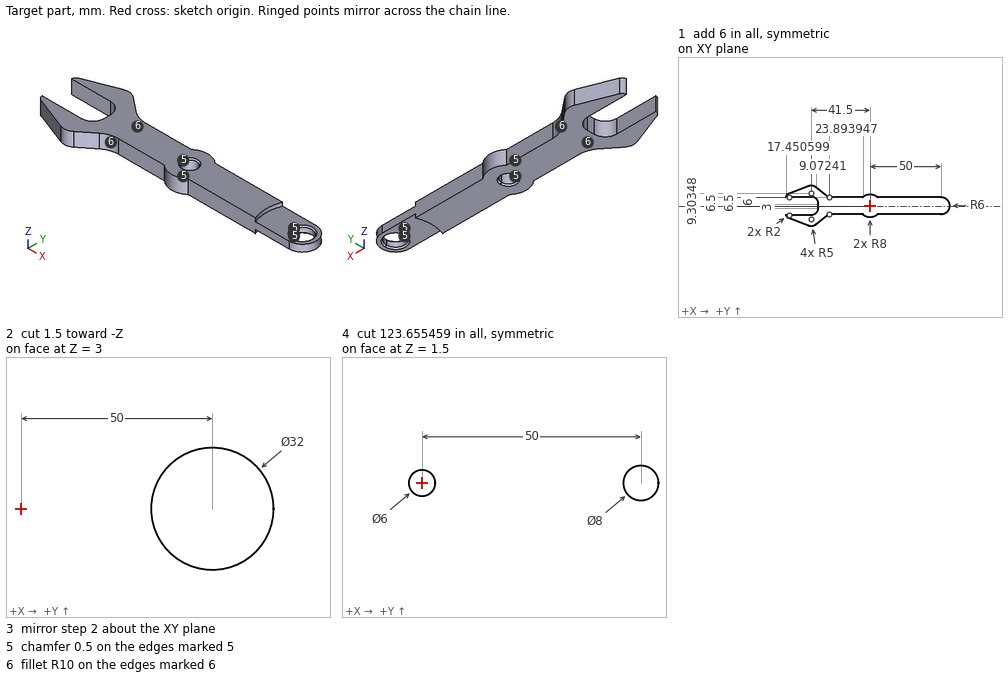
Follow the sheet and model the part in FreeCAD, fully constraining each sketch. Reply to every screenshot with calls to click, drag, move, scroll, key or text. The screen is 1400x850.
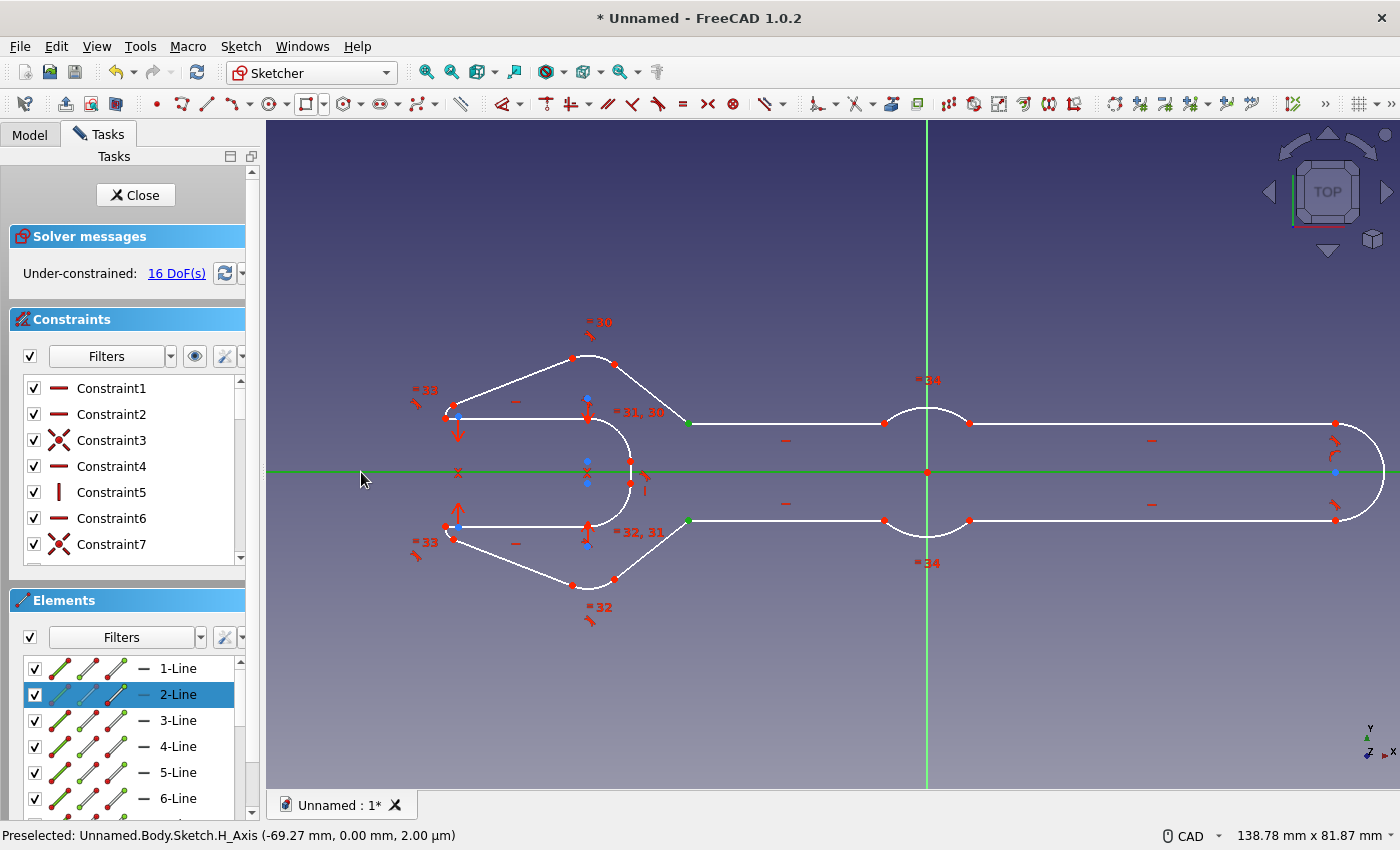
click(708, 104)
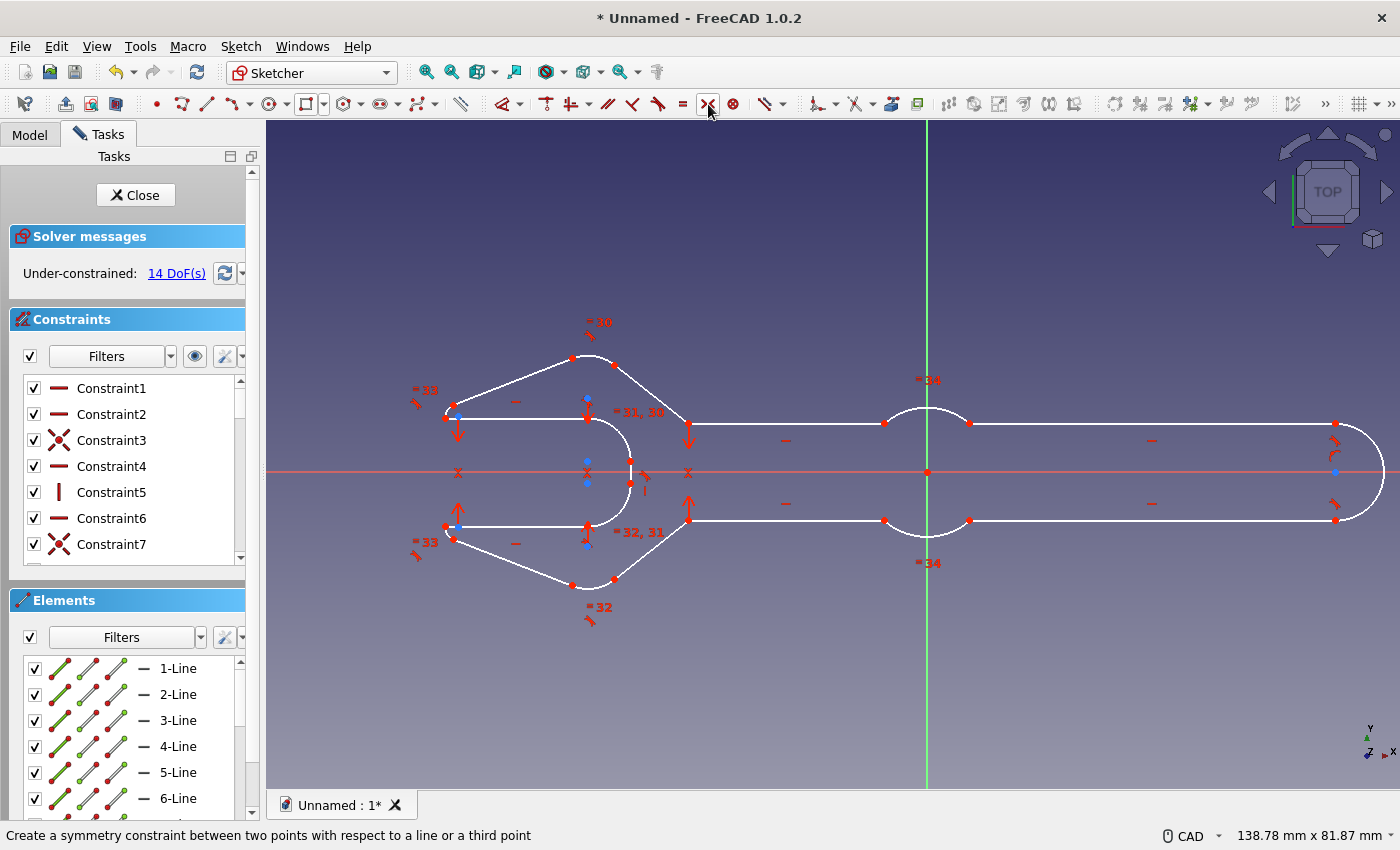
click(502, 104)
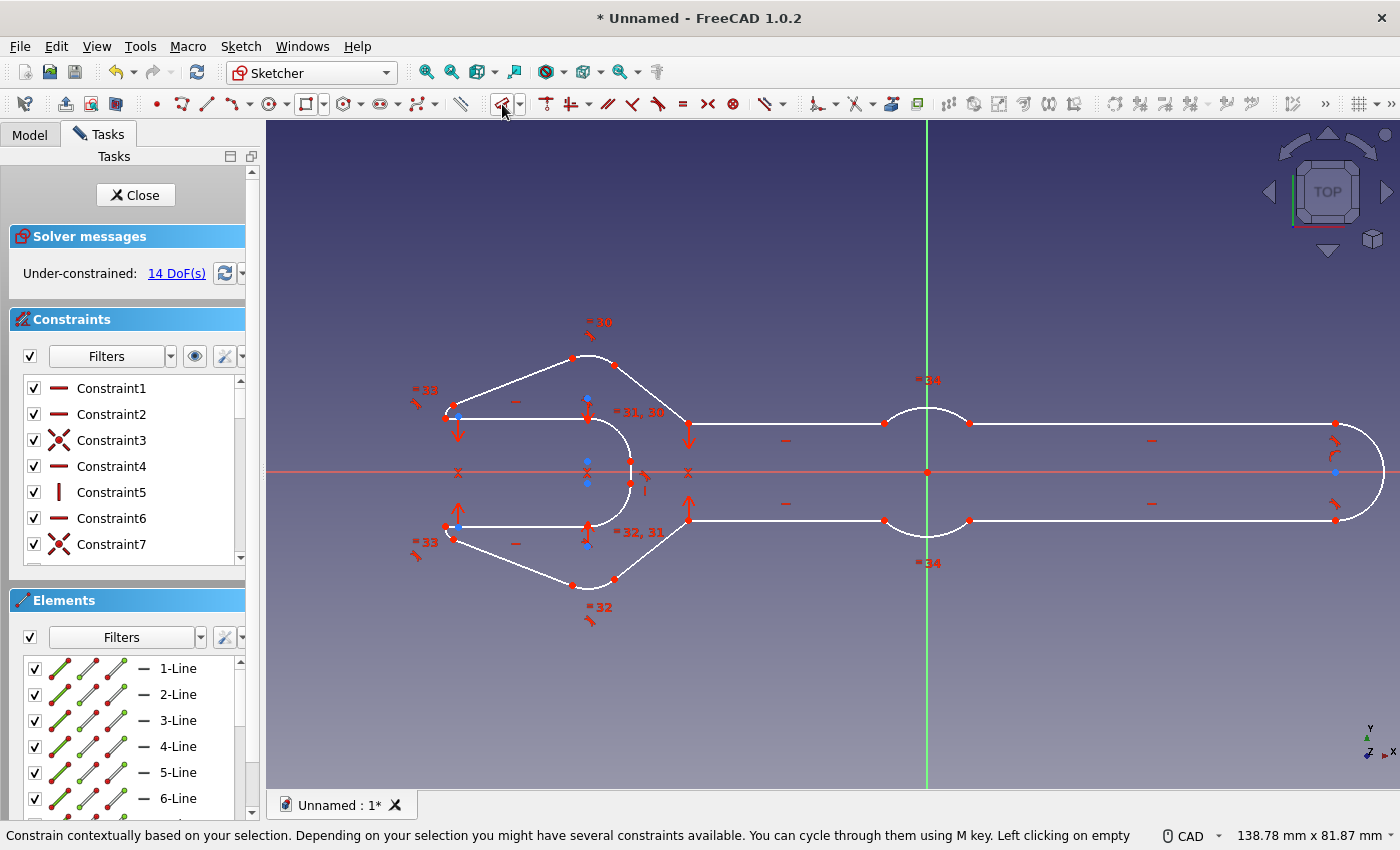
click(945, 410)
click(954, 379)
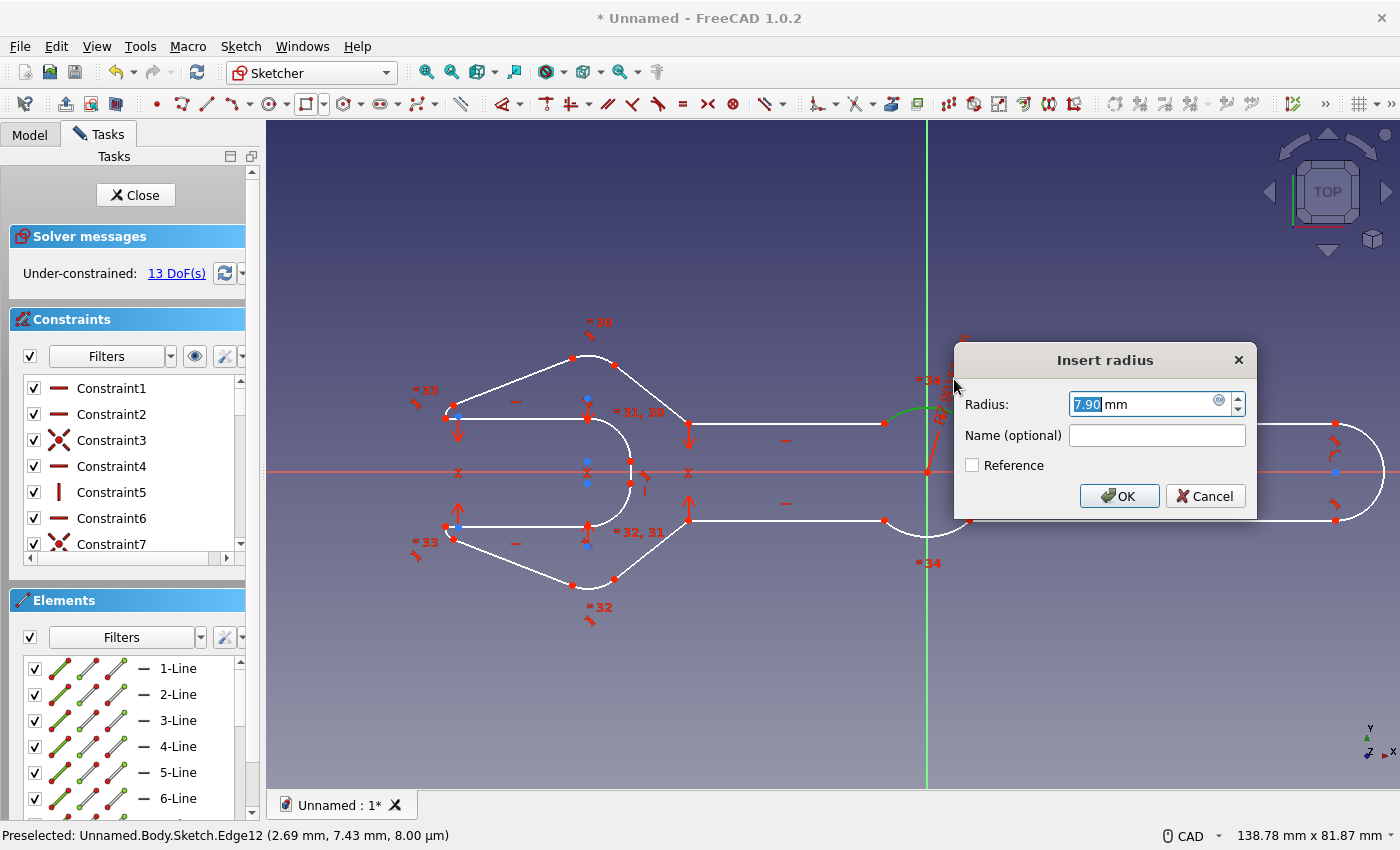
text(8)
key(Return)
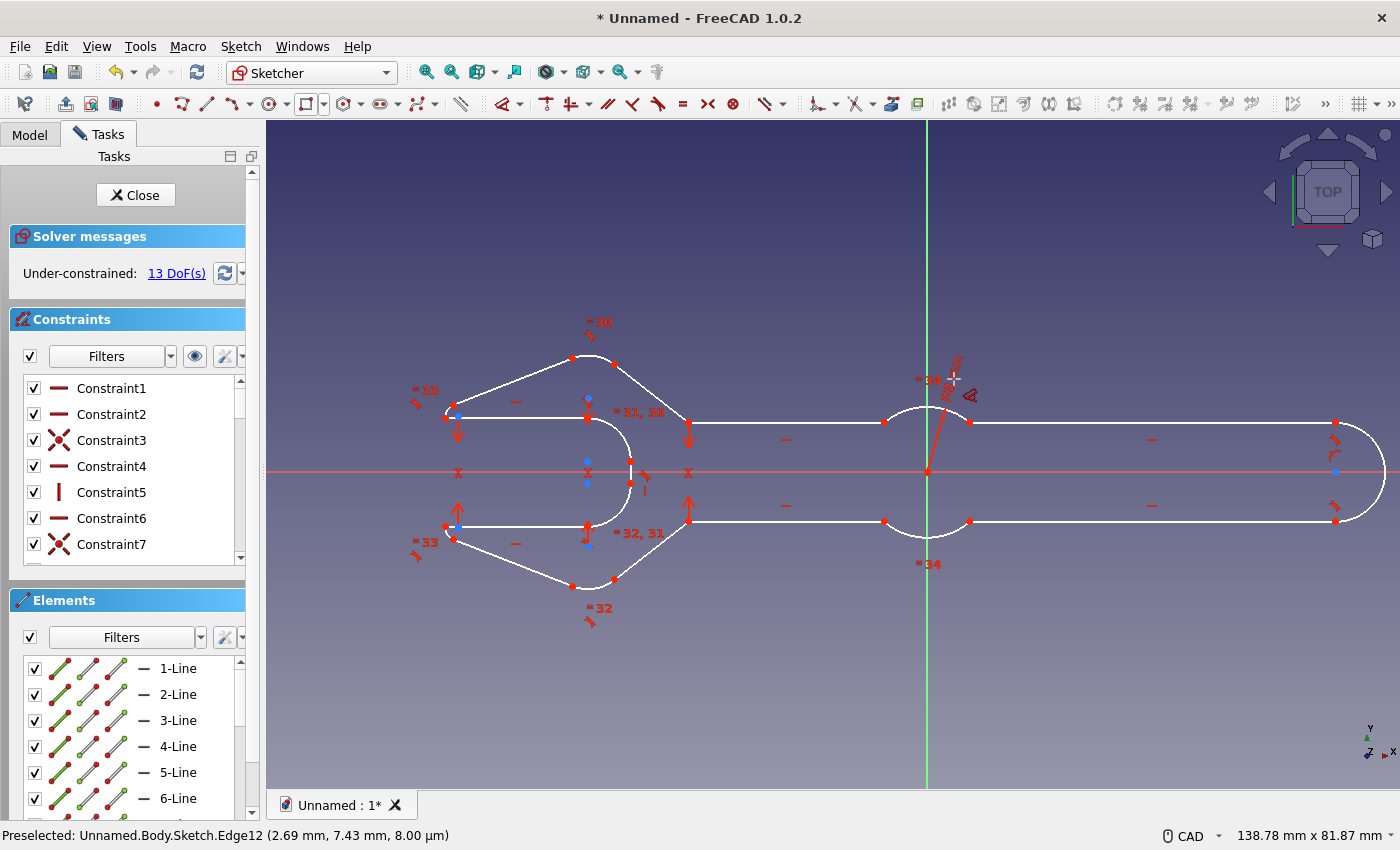
click(603, 358)
click(614, 328)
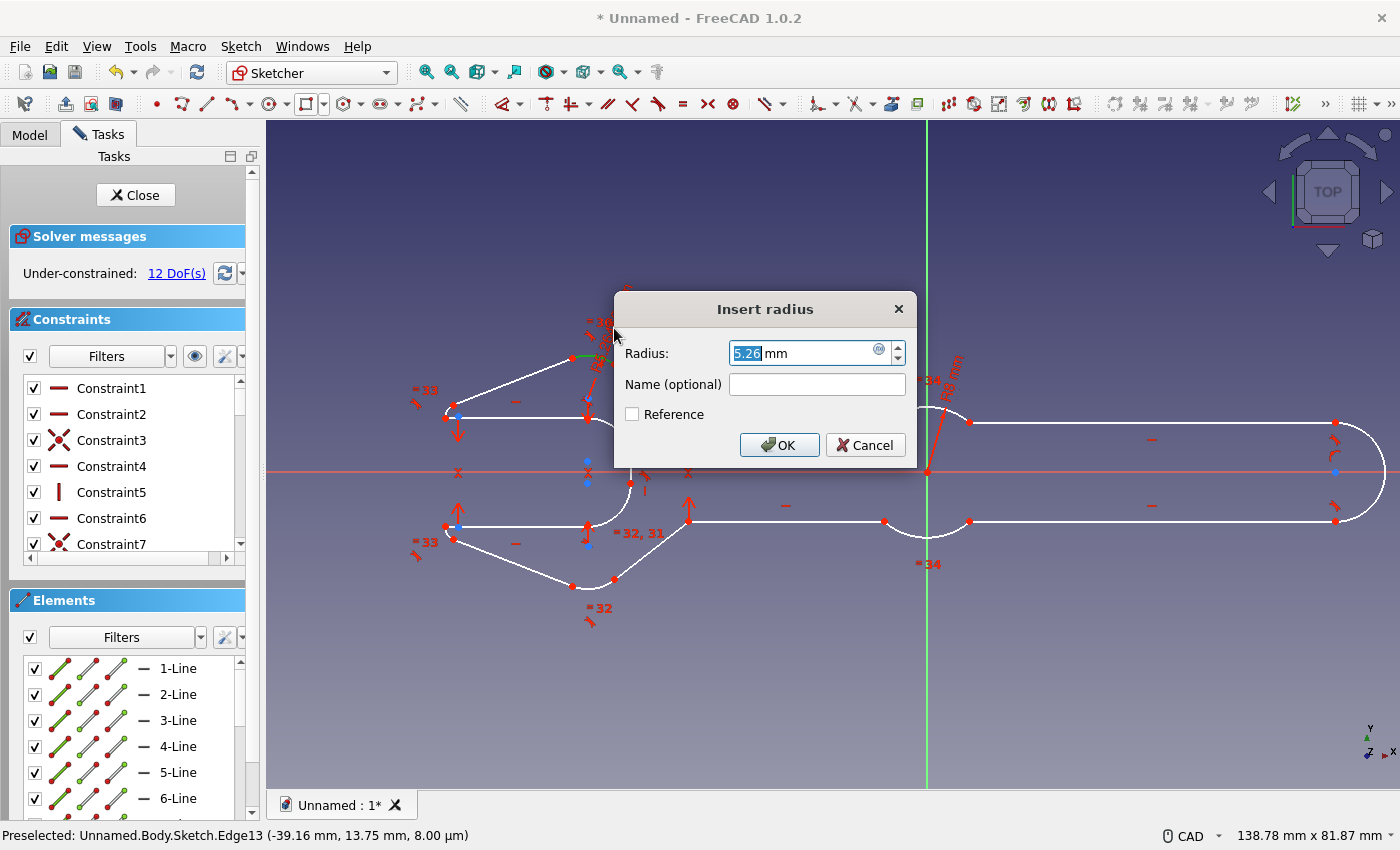
text(5)
key(Return)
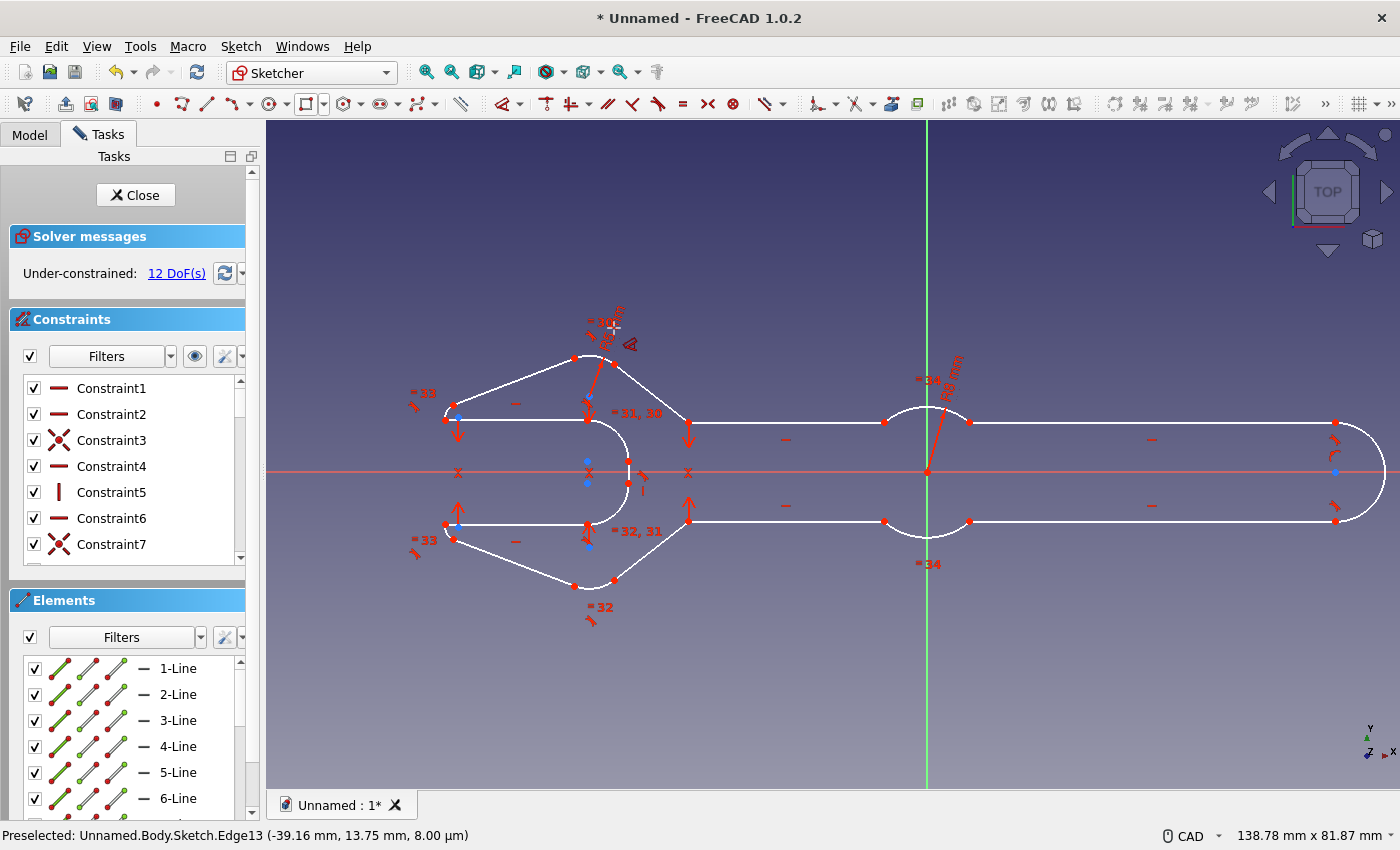
scroll(447, 411, up, 5)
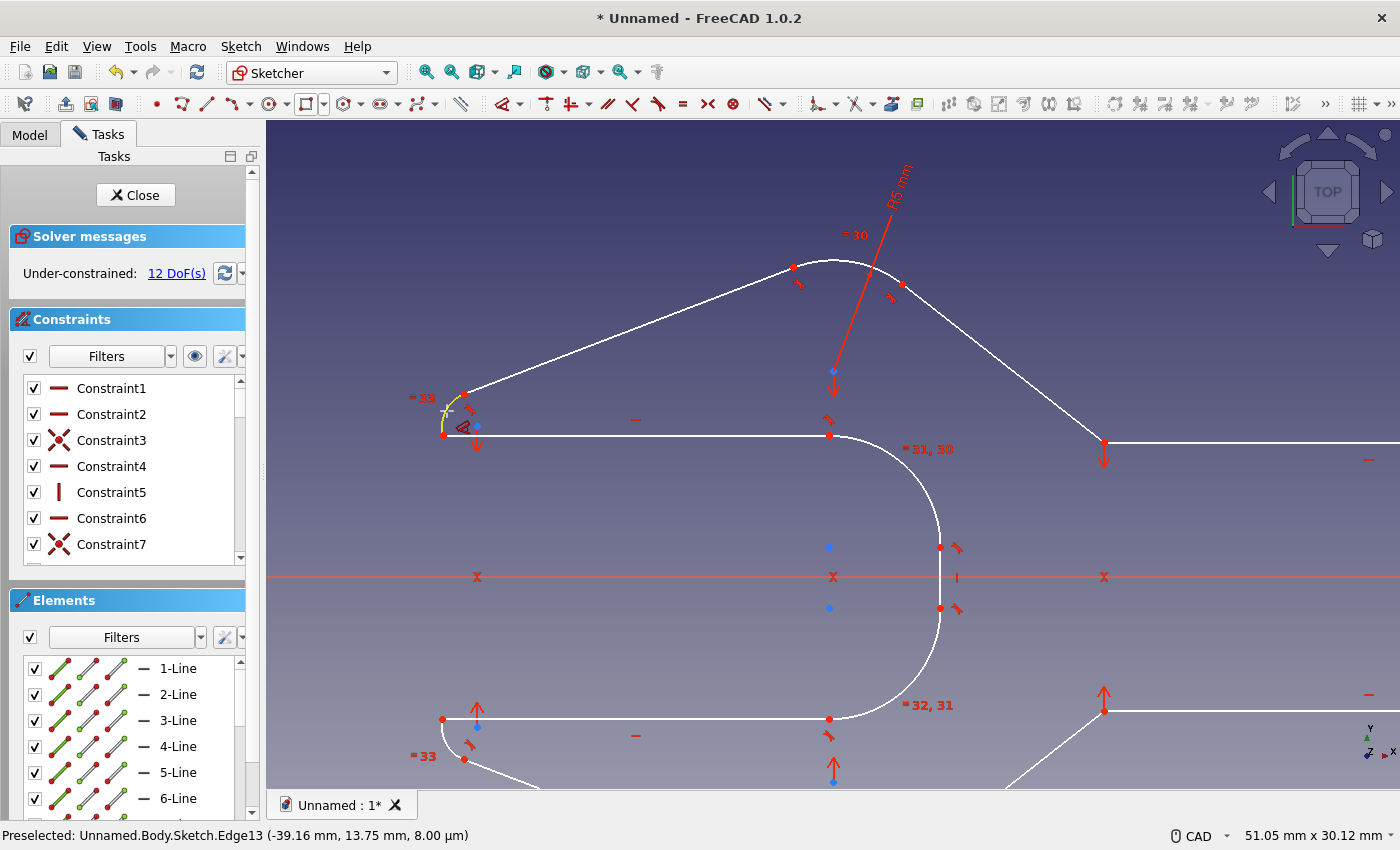
click(446, 411)
click(417, 396)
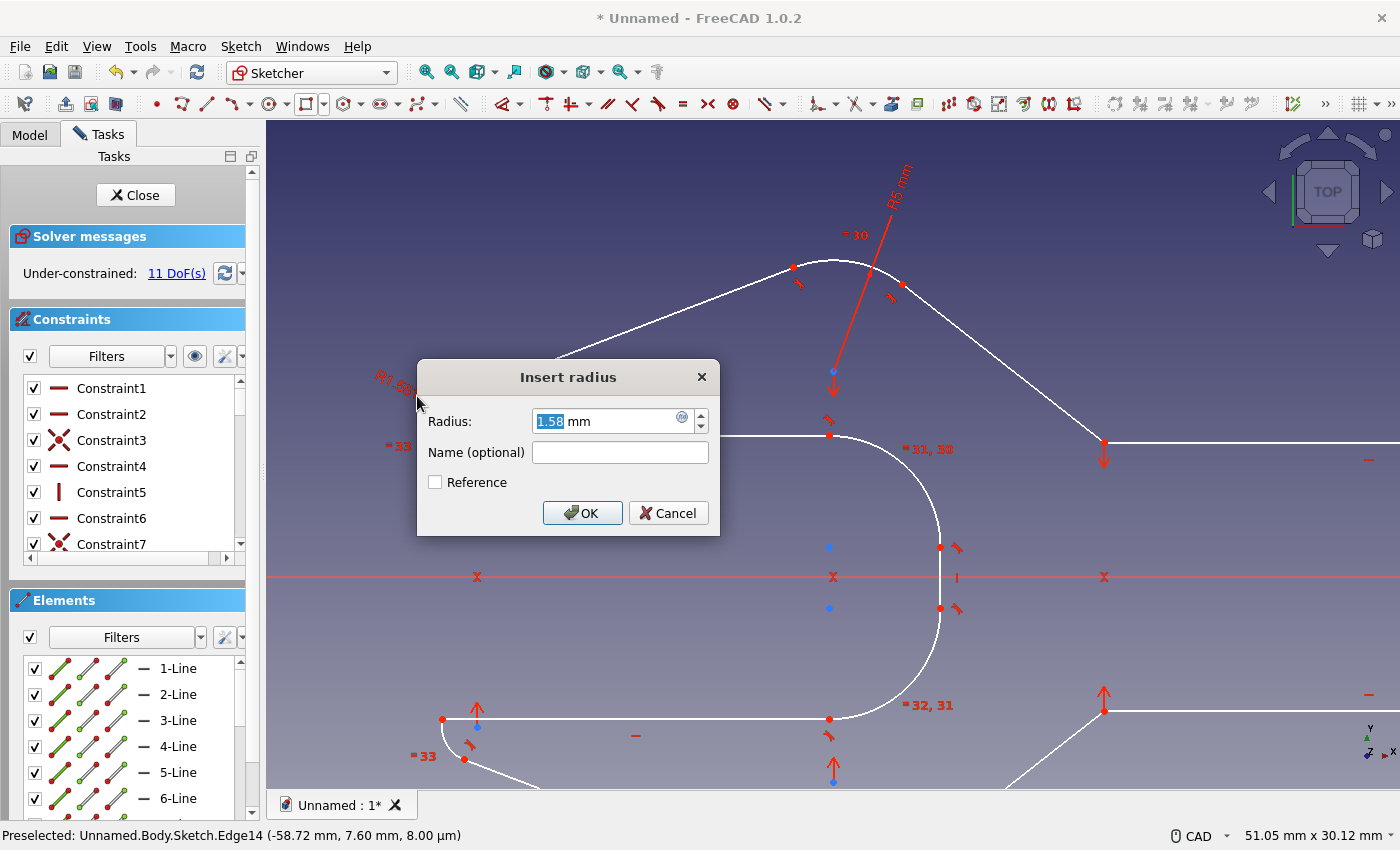
text(2)
key(Return)